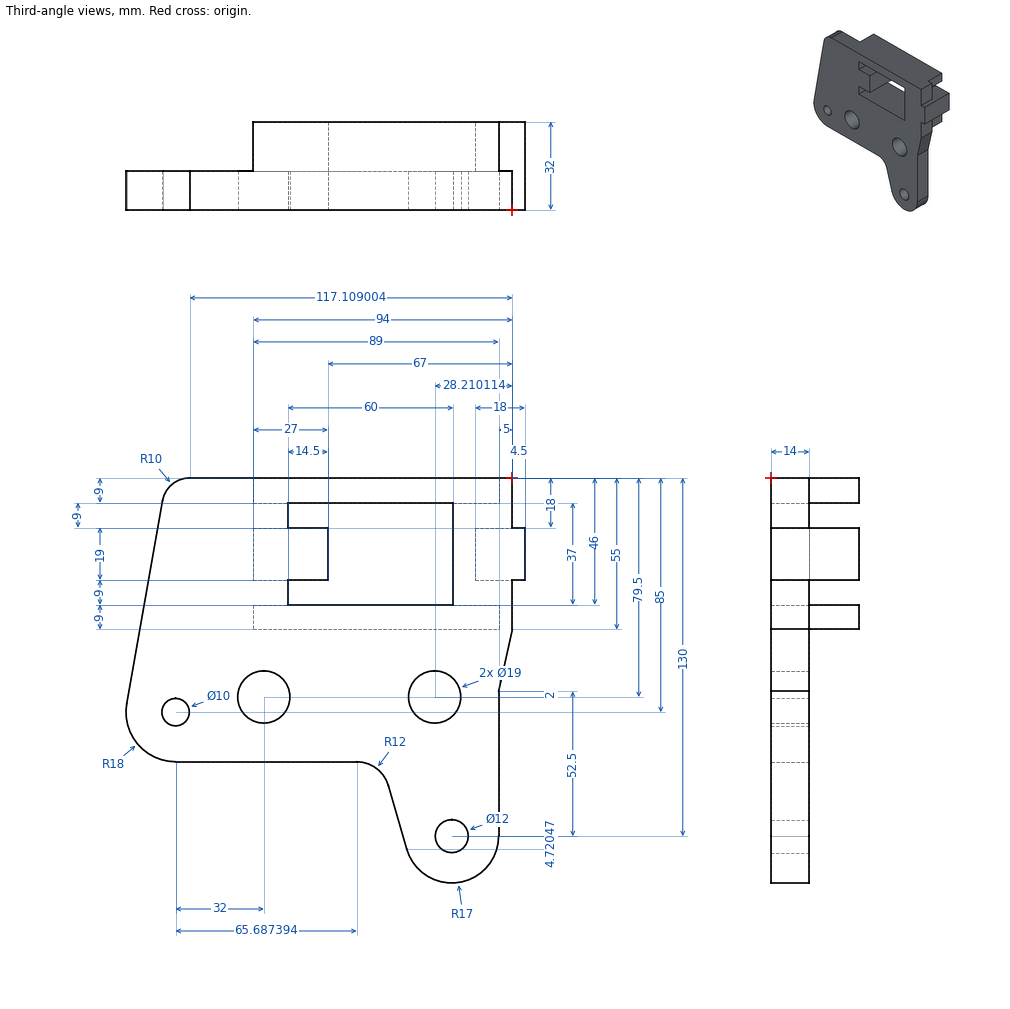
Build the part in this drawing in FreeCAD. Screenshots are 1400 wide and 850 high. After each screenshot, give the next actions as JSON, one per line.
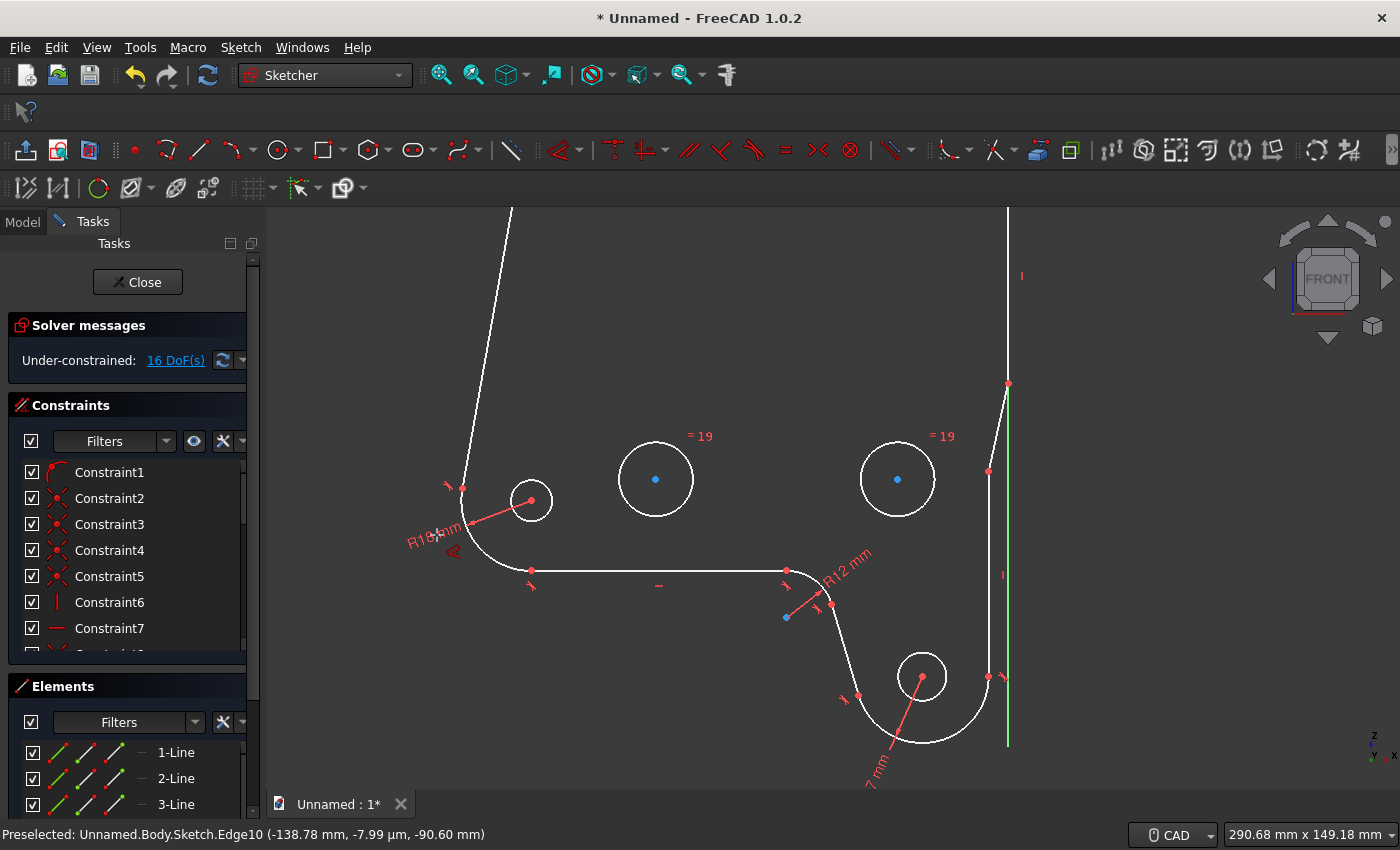
{"action": "scroll", "coordinate": [824, 587], "scroll_direction": "down", "scroll_amount": 2}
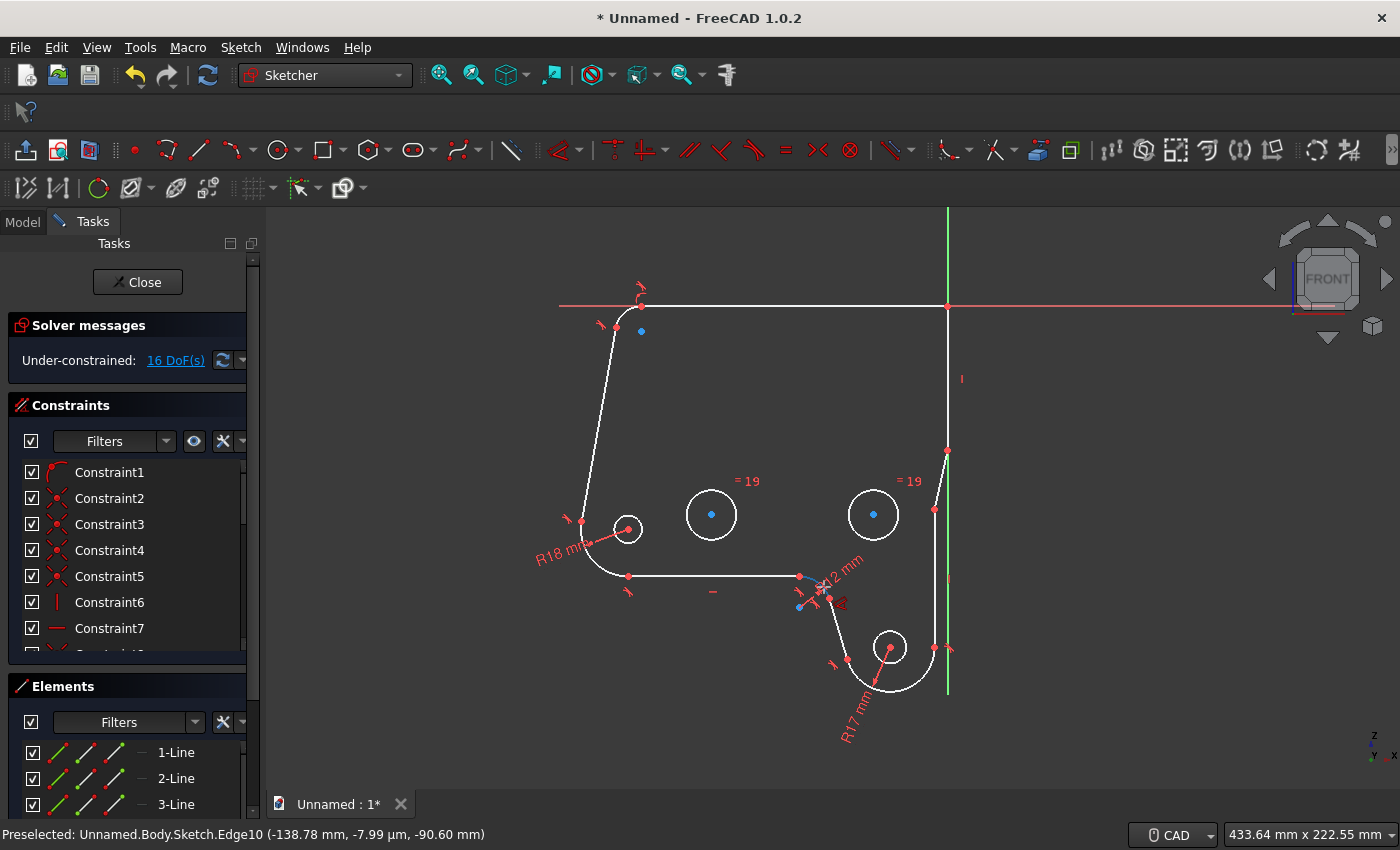
{"action": "scroll", "coordinate": [631, 309], "scroll_direction": "up", "scroll_amount": 3}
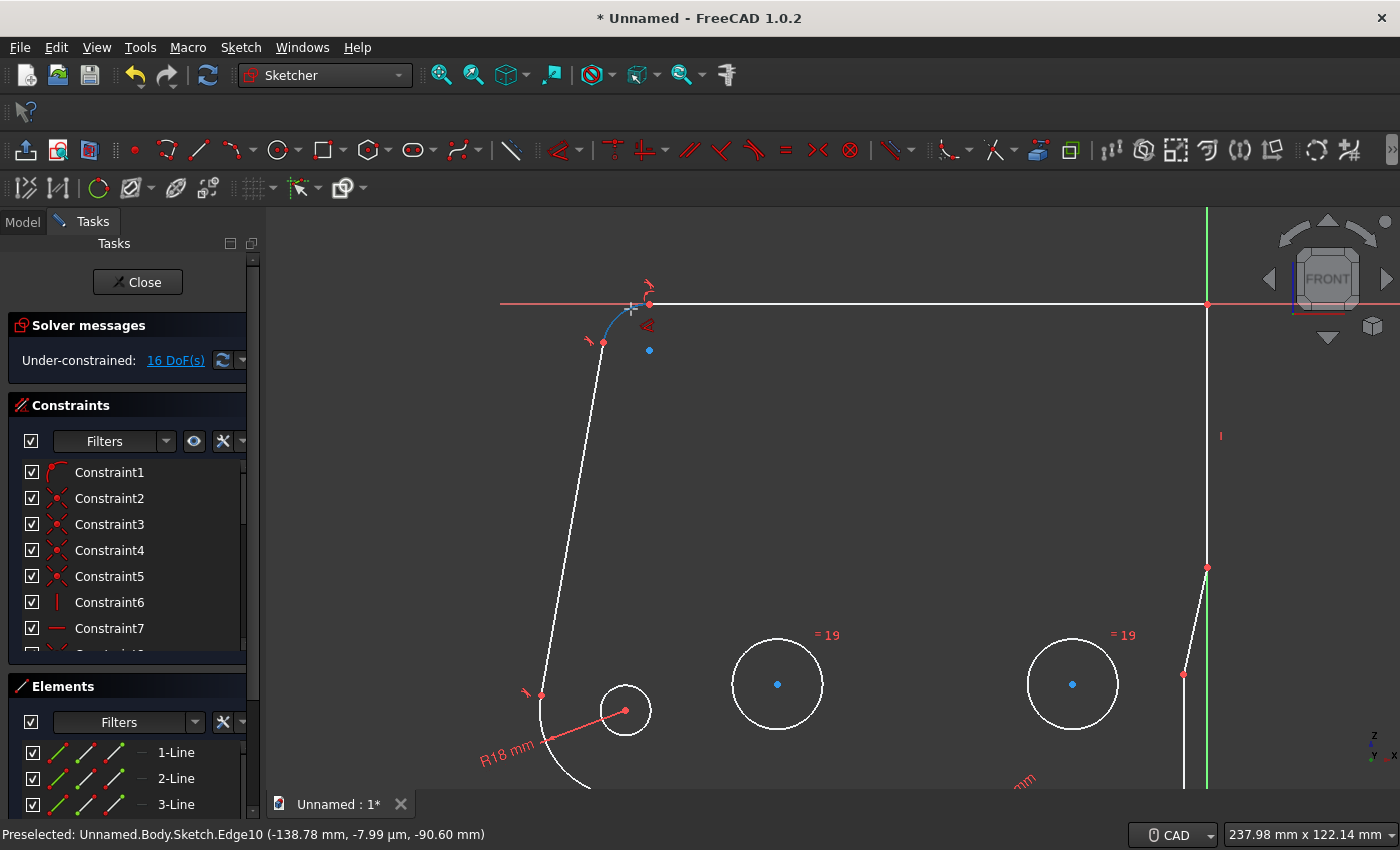
{"action": "left_click", "coordinate": [630, 308]}
{"action": "left_click", "coordinate": [617, 279]}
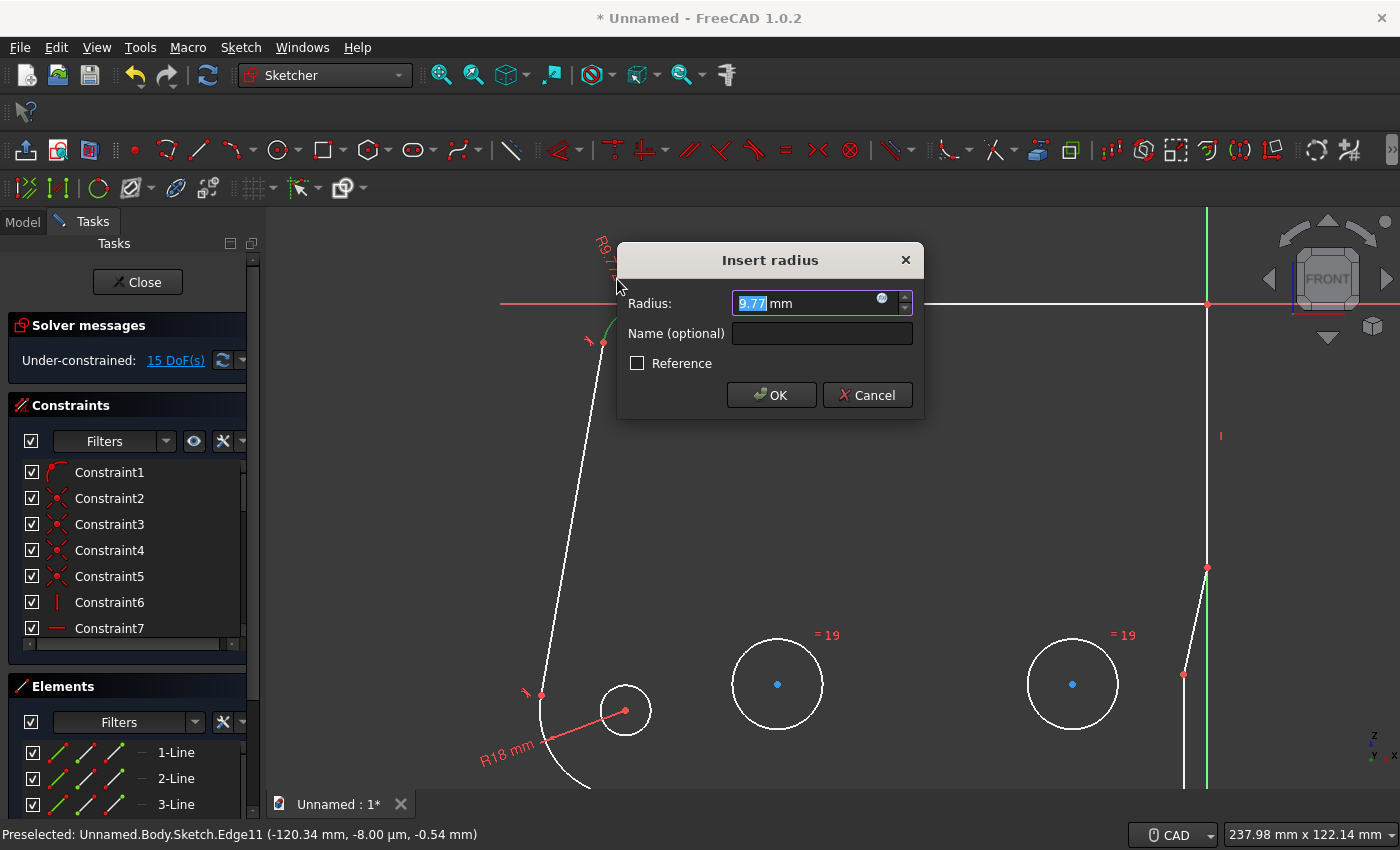
{"action": "type", "text": "10"}
{"action": "key", "text": "Return"}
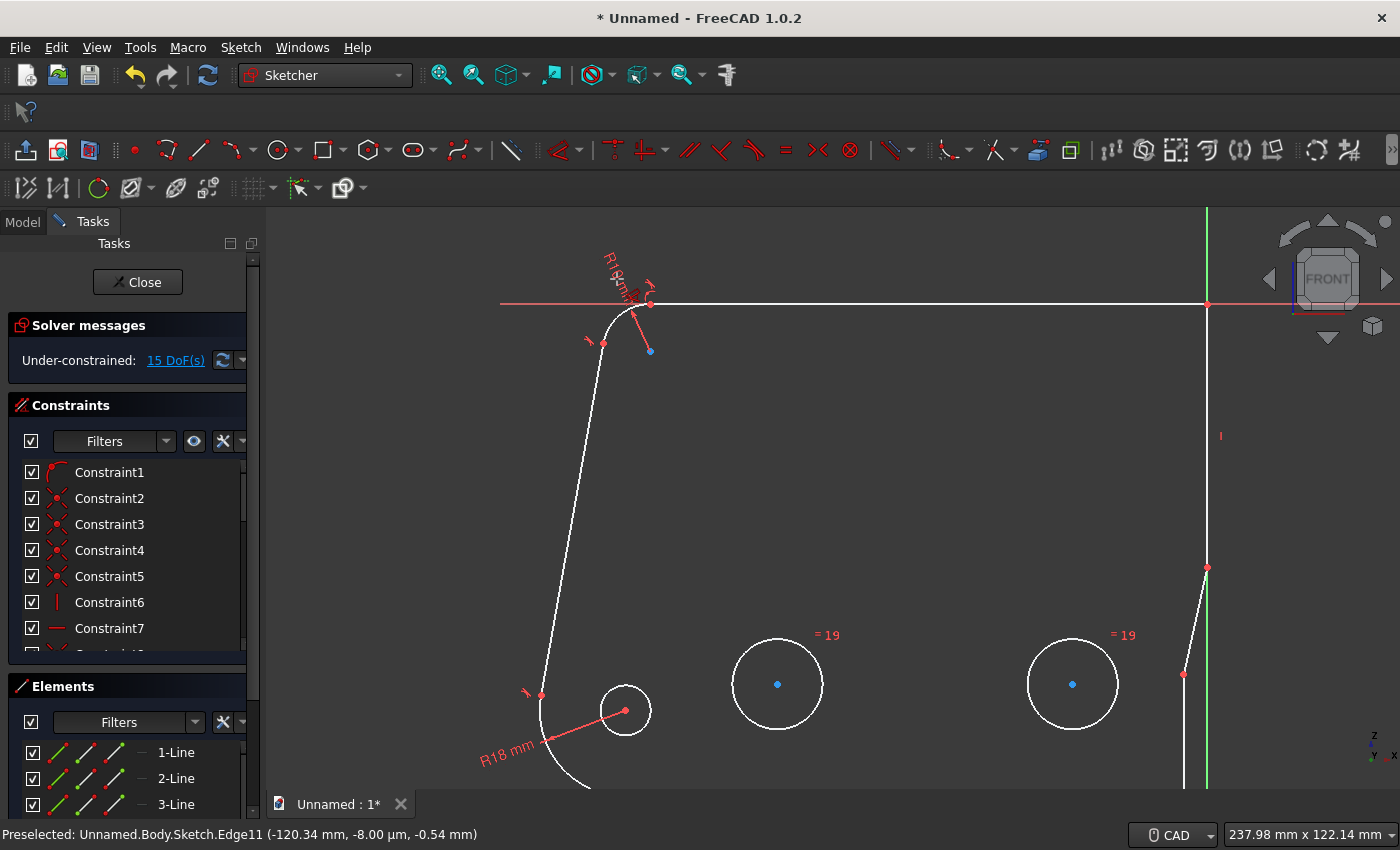
{"action": "left_click", "coordinate": [1104, 652]}
{"action": "left_click", "coordinate": [1126, 629]}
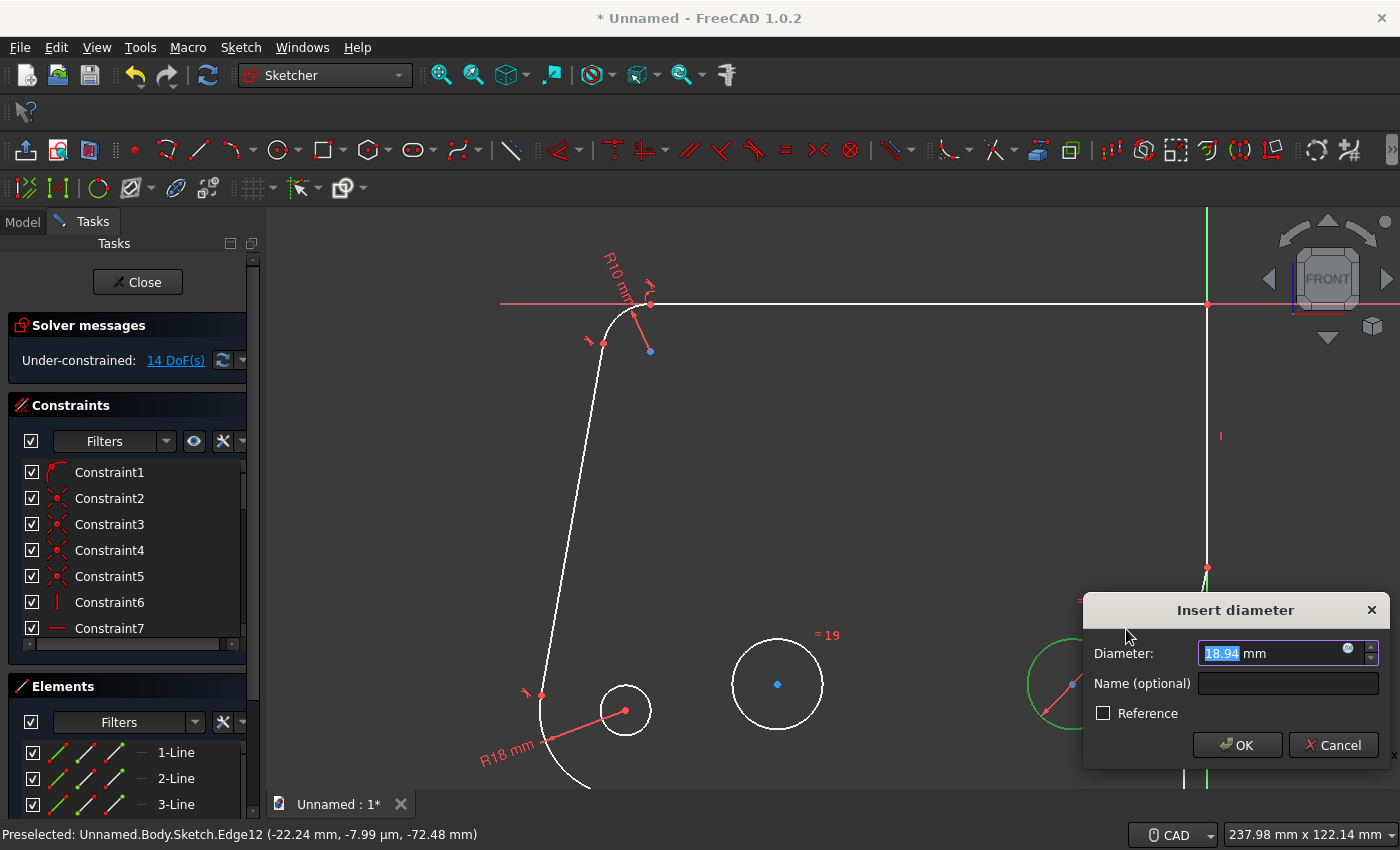
{"action": "type", "text": "19"}
{"action": "key", "text": "Return"}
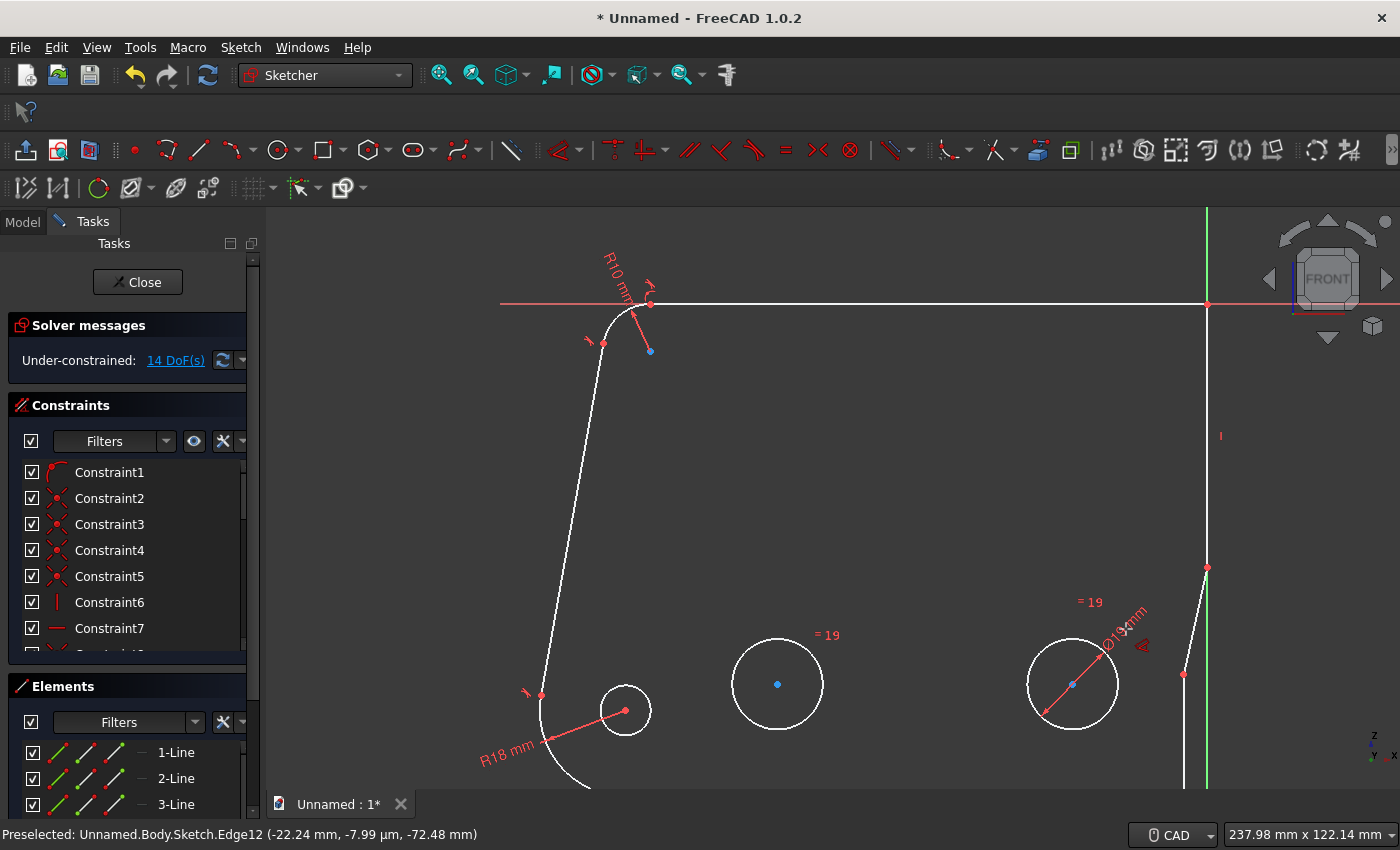
{"action": "left_click", "coordinate": [643, 693]}
{"action": "left_click", "coordinate": [666, 670]}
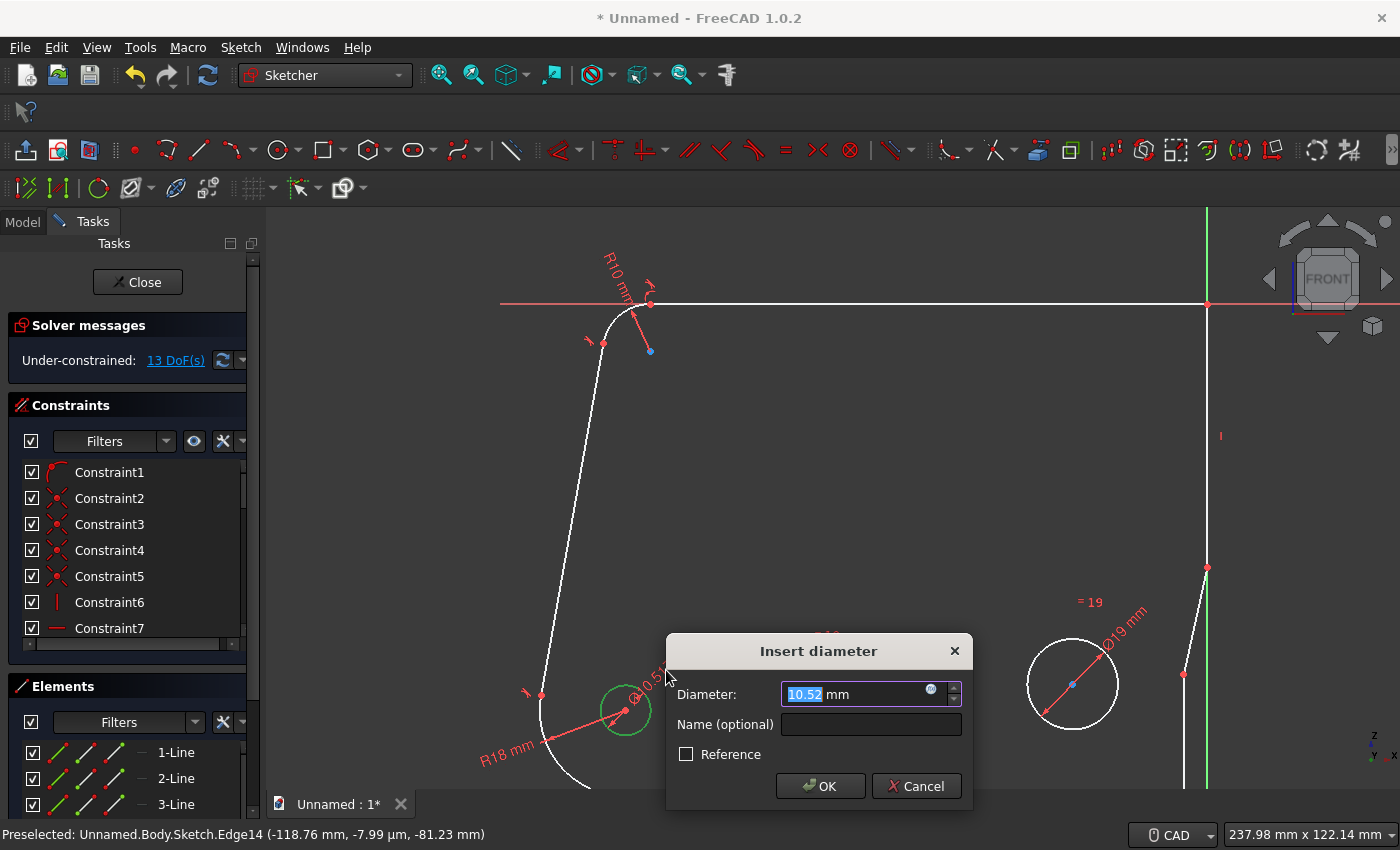
{"action": "type", "text": "10"}
{"action": "key", "text": "Return"}